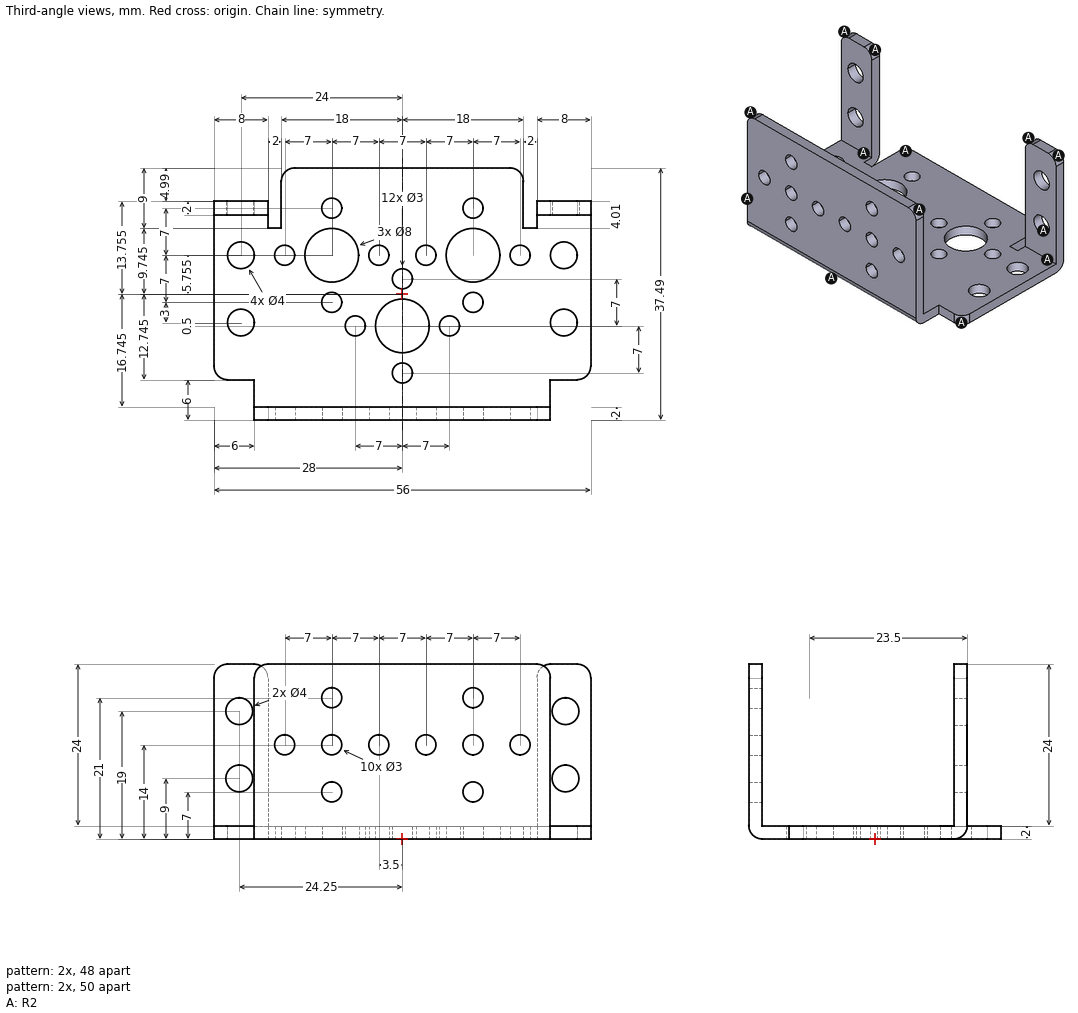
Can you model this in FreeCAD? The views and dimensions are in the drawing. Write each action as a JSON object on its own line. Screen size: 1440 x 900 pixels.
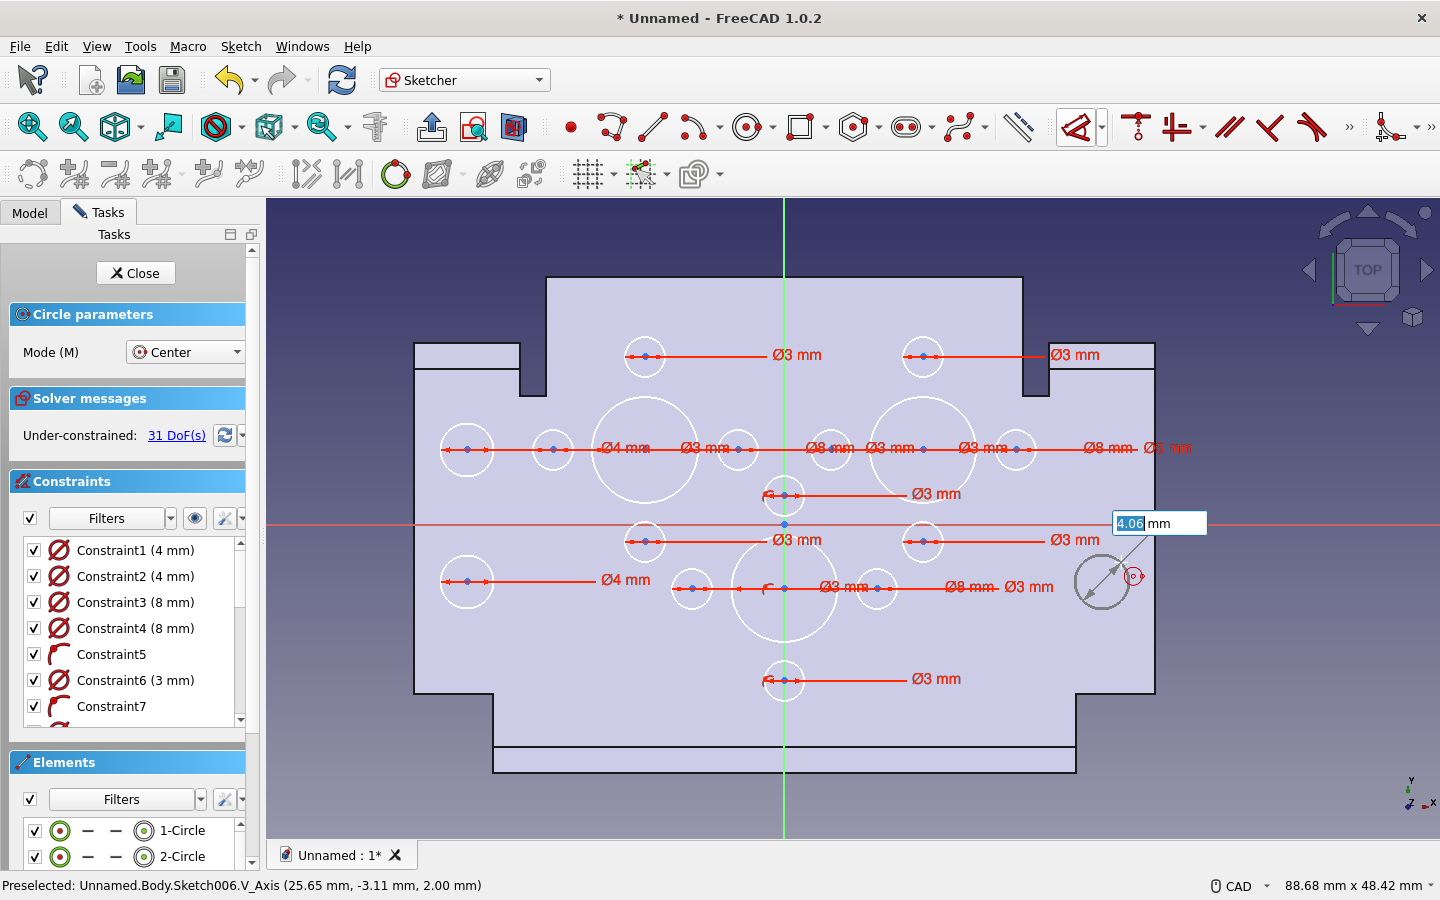
{"action": "type", "text": "4"}
{"action": "key", "text": "Return"}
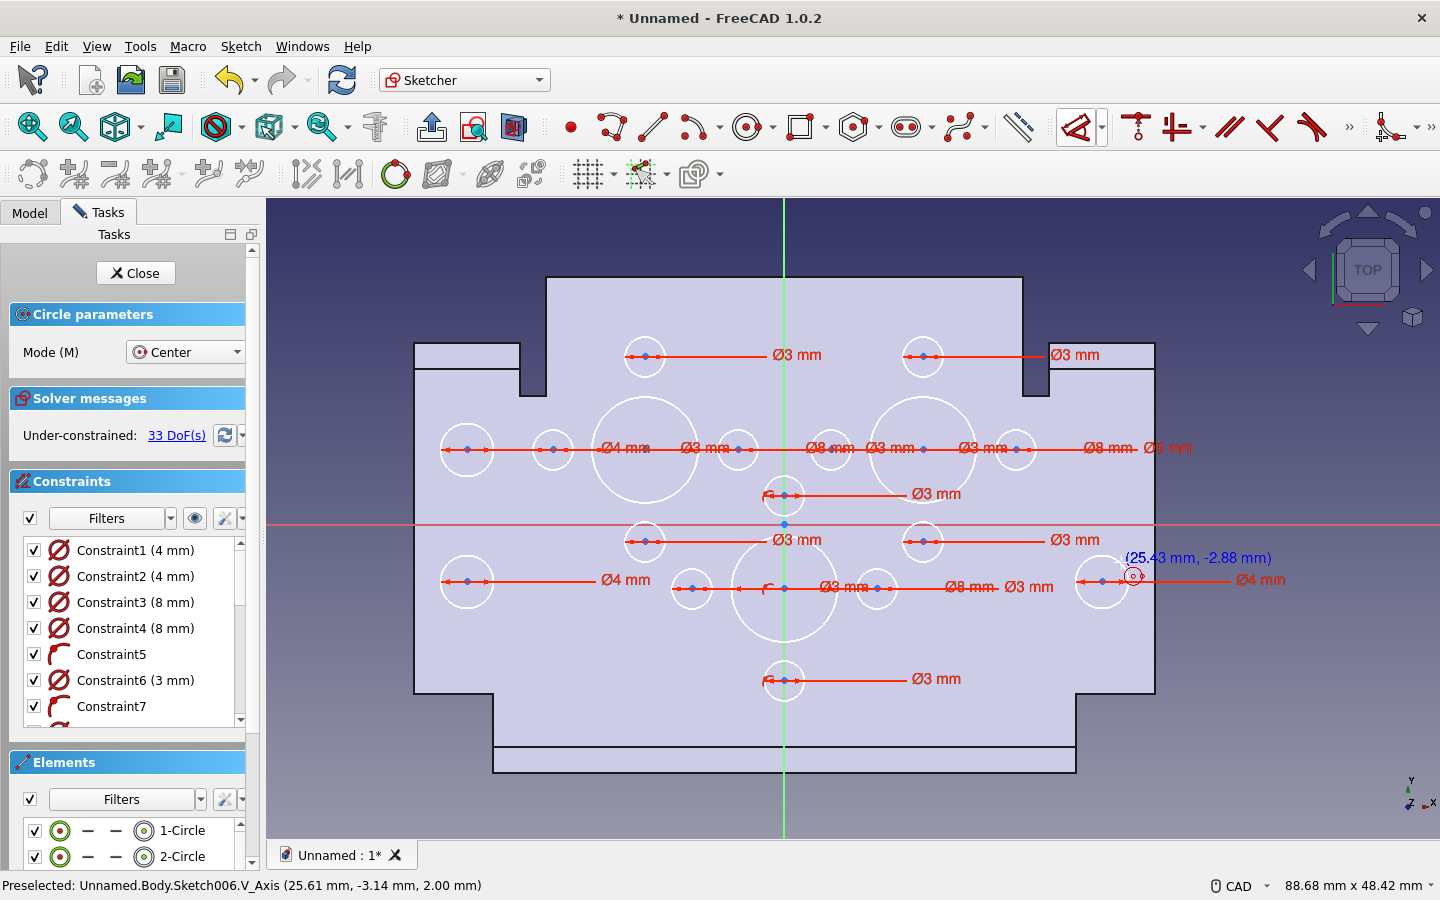
{"action": "left_click", "coordinate": [1102, 449]}
{"action": "mouse_move", "coordinate": [1121, 430]}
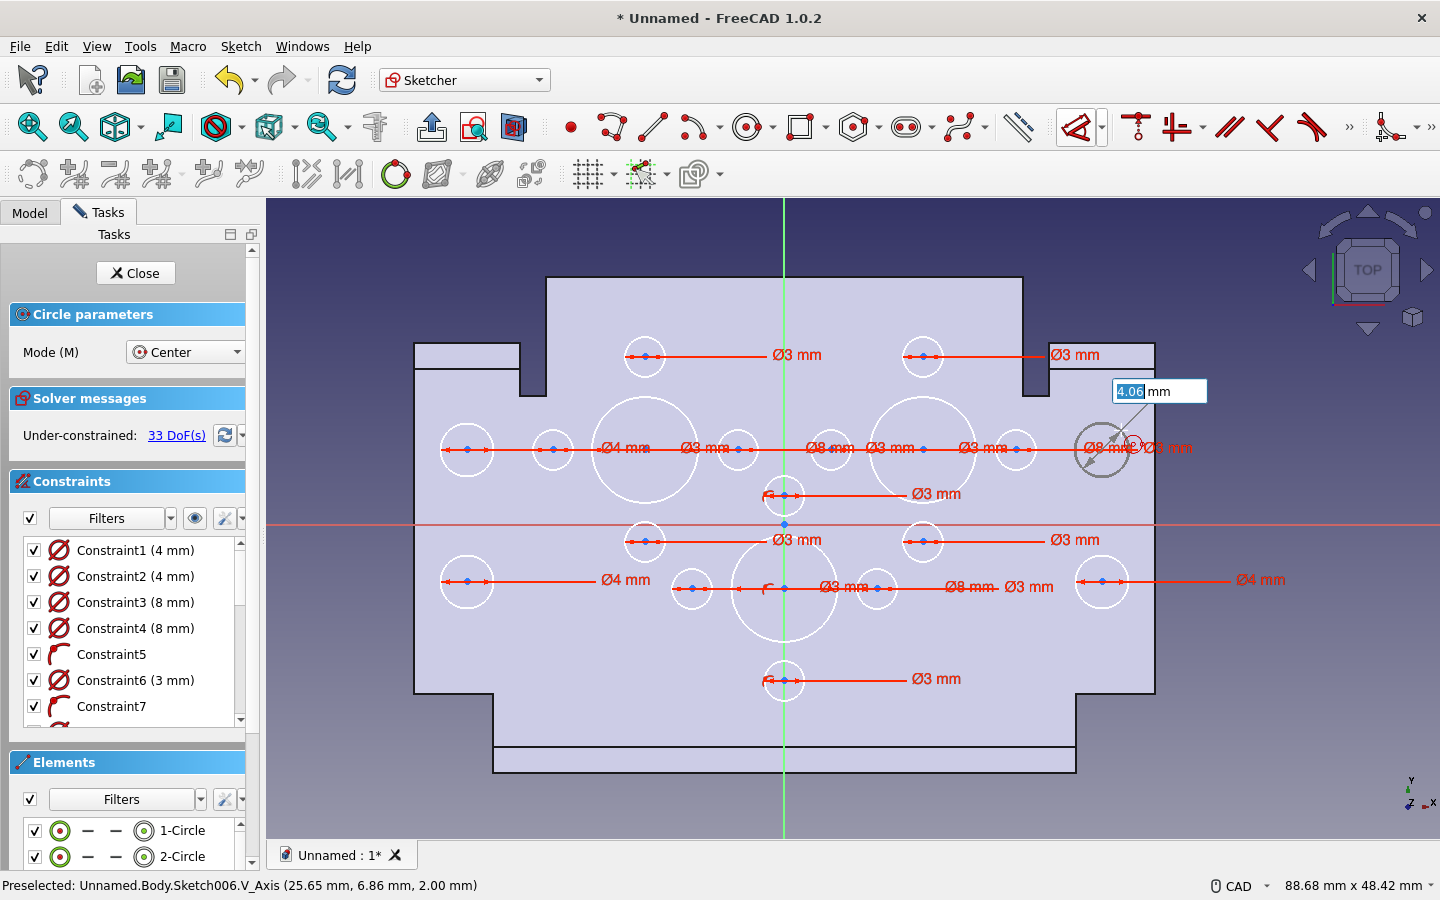
{"action": "type", "text": "4"}
{"action": "key", "text": "Return"}
{"action": "key", "text": "Escape"}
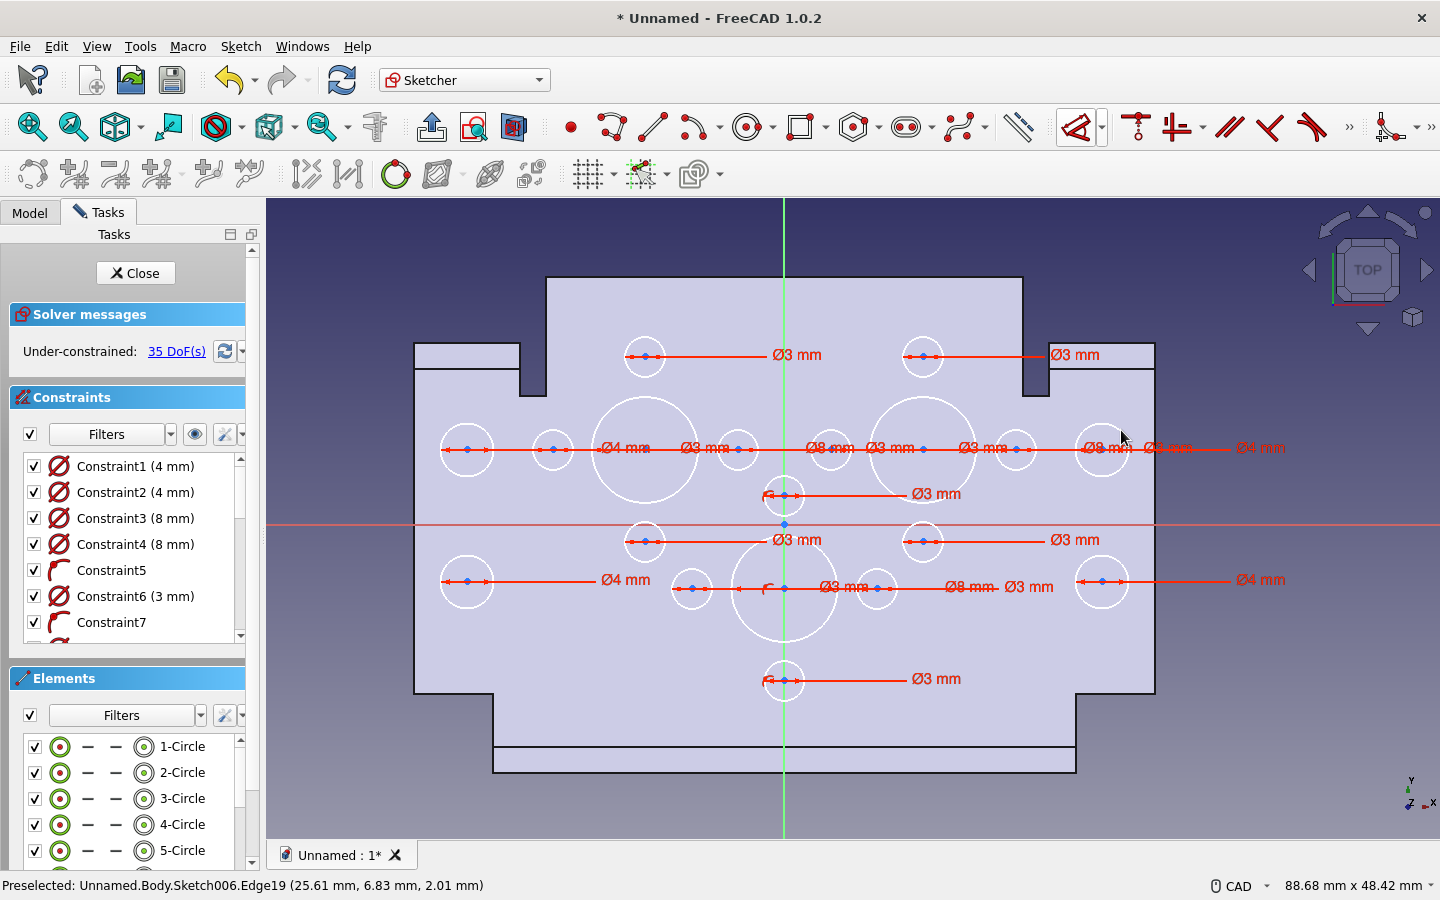
{"action": "left_click", "coordinate": [467, 450]}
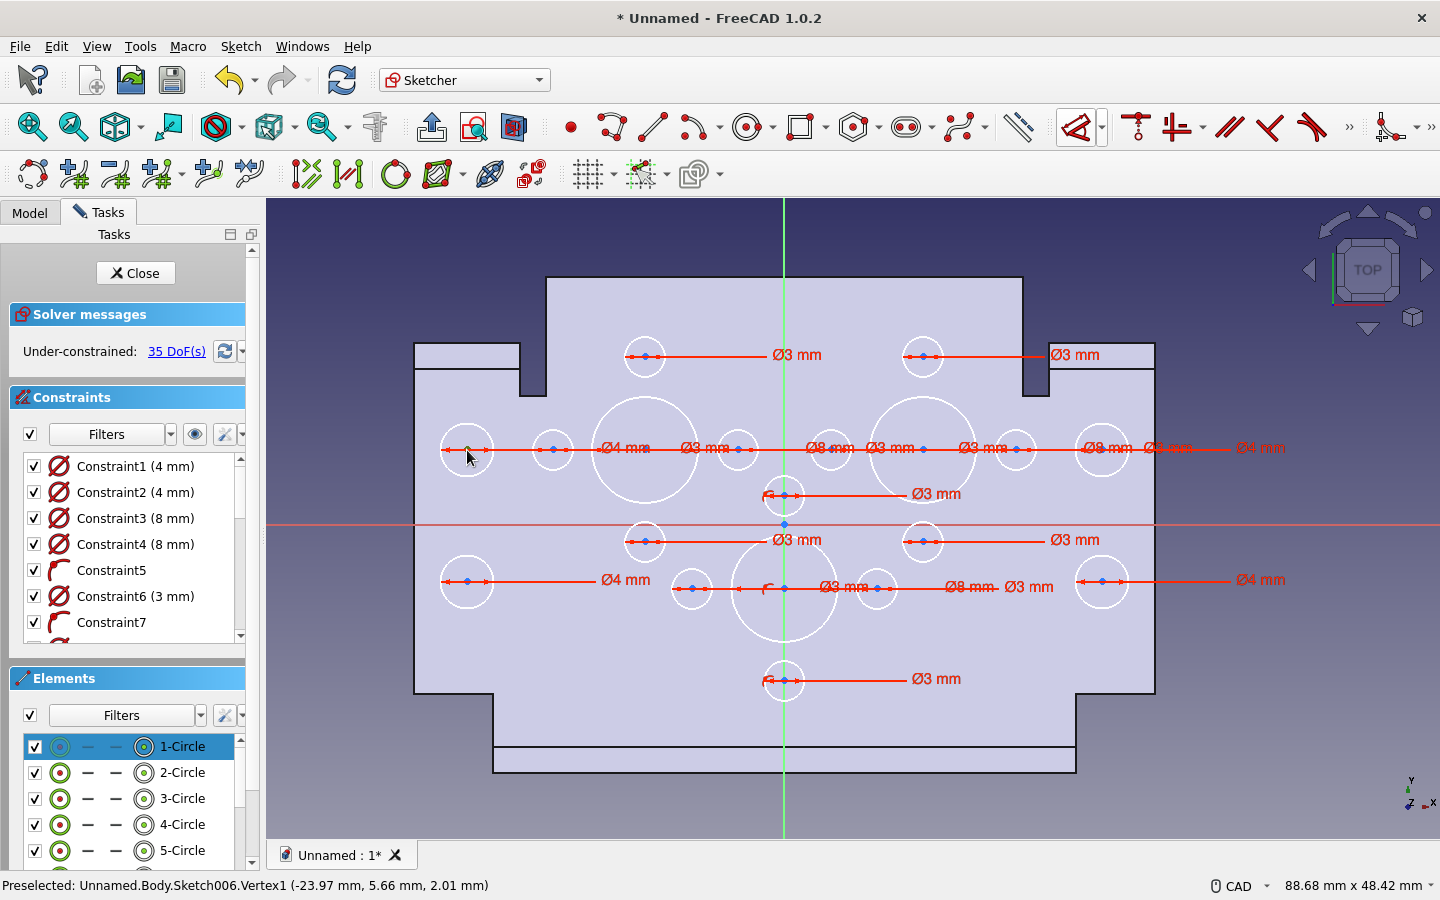
{"action": "left_click", "coordinate": [467, 582]}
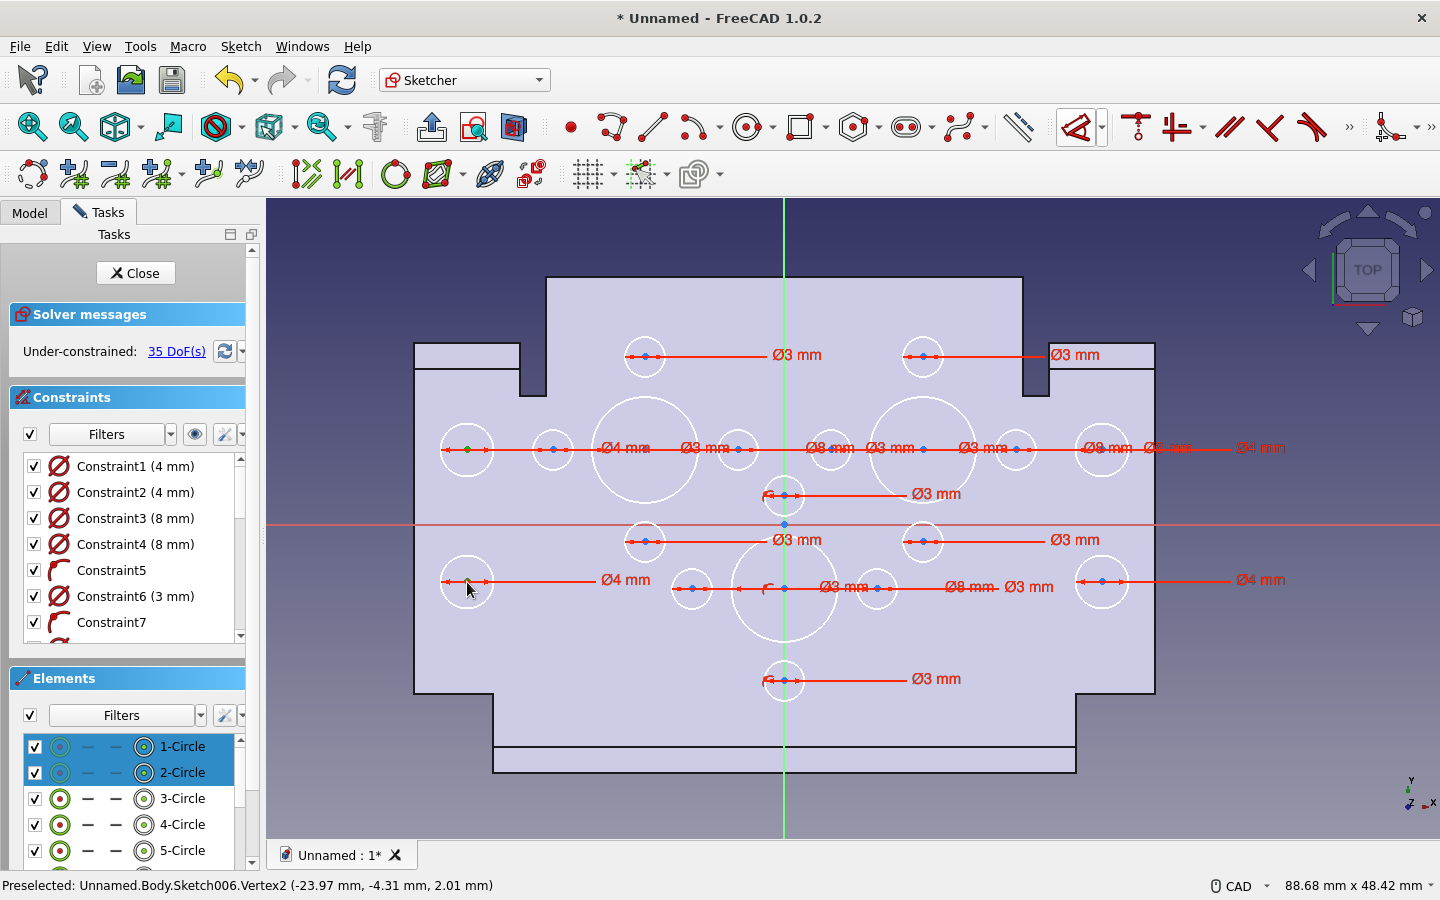
{"action": "key", "text": "v"}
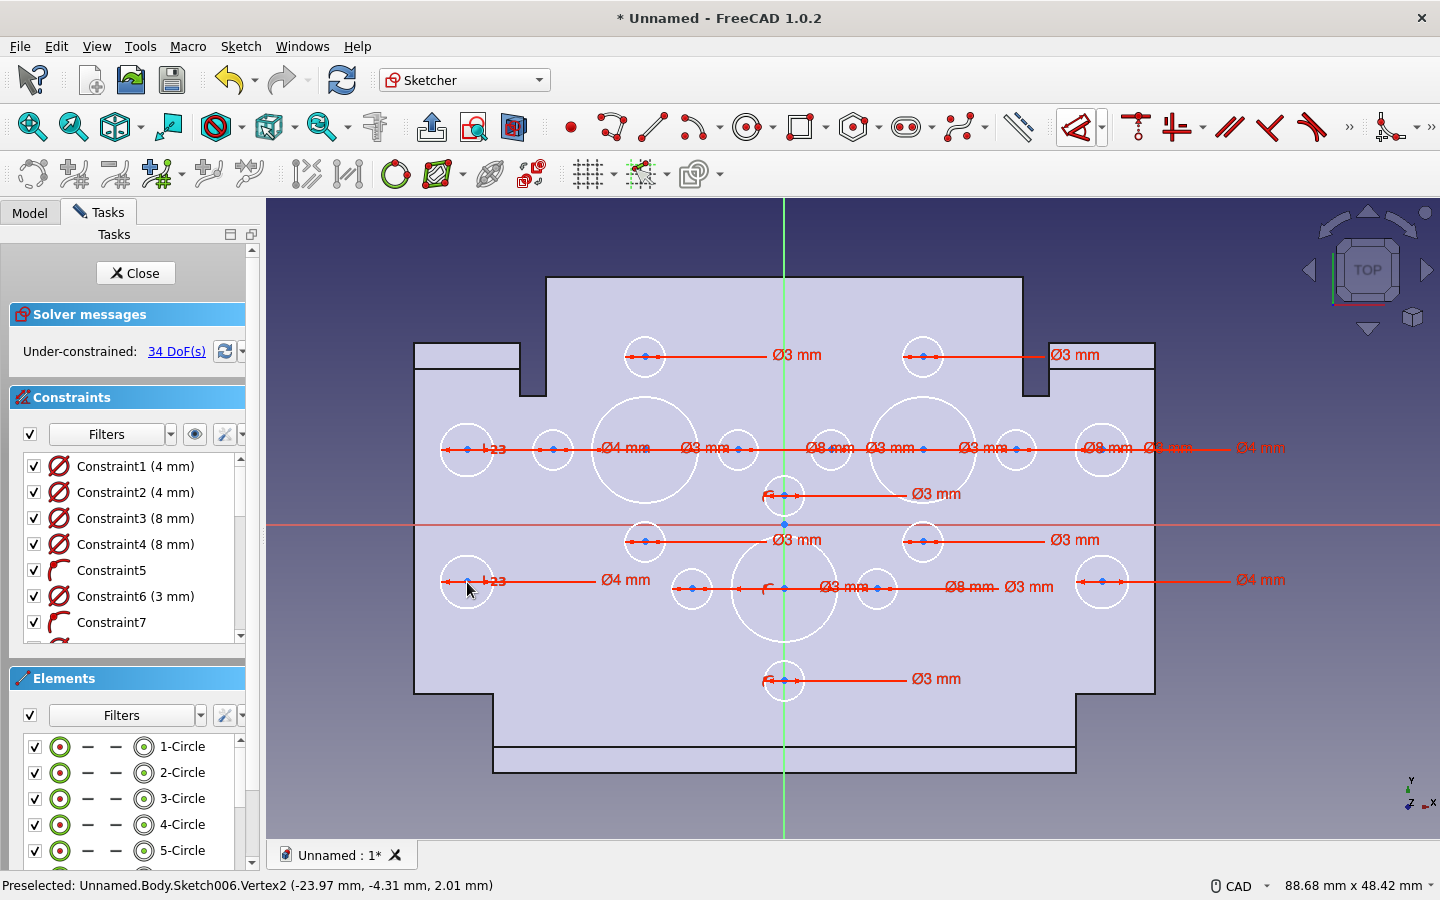
{"action": "left_click", "coordinate": [467, 450]}